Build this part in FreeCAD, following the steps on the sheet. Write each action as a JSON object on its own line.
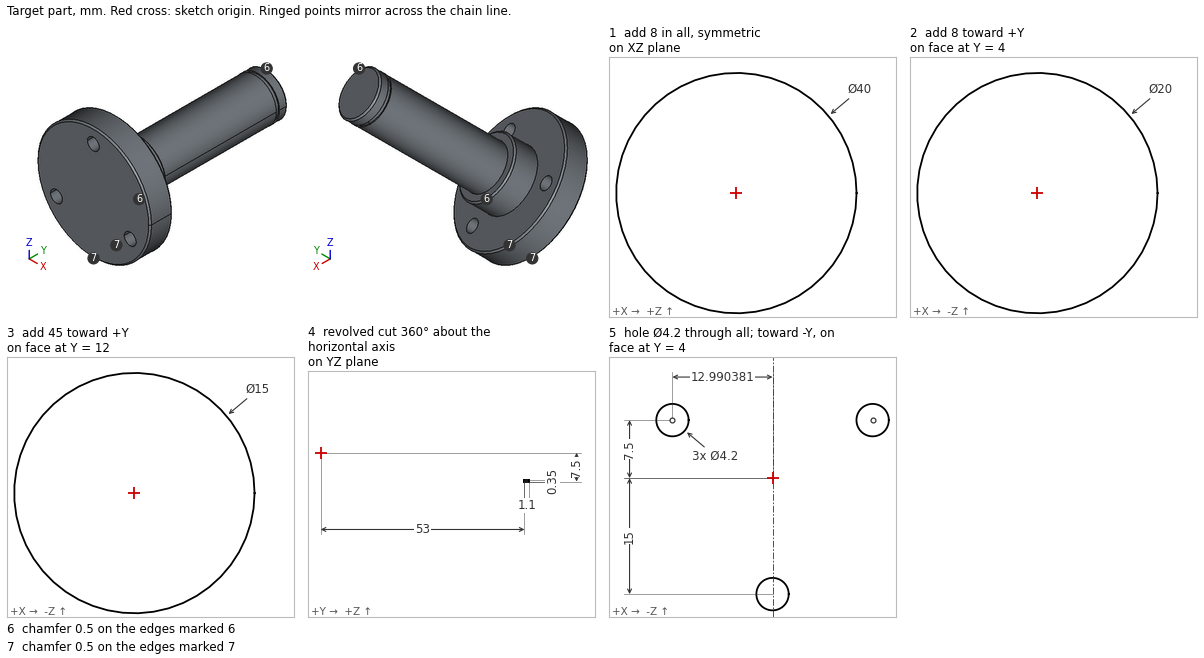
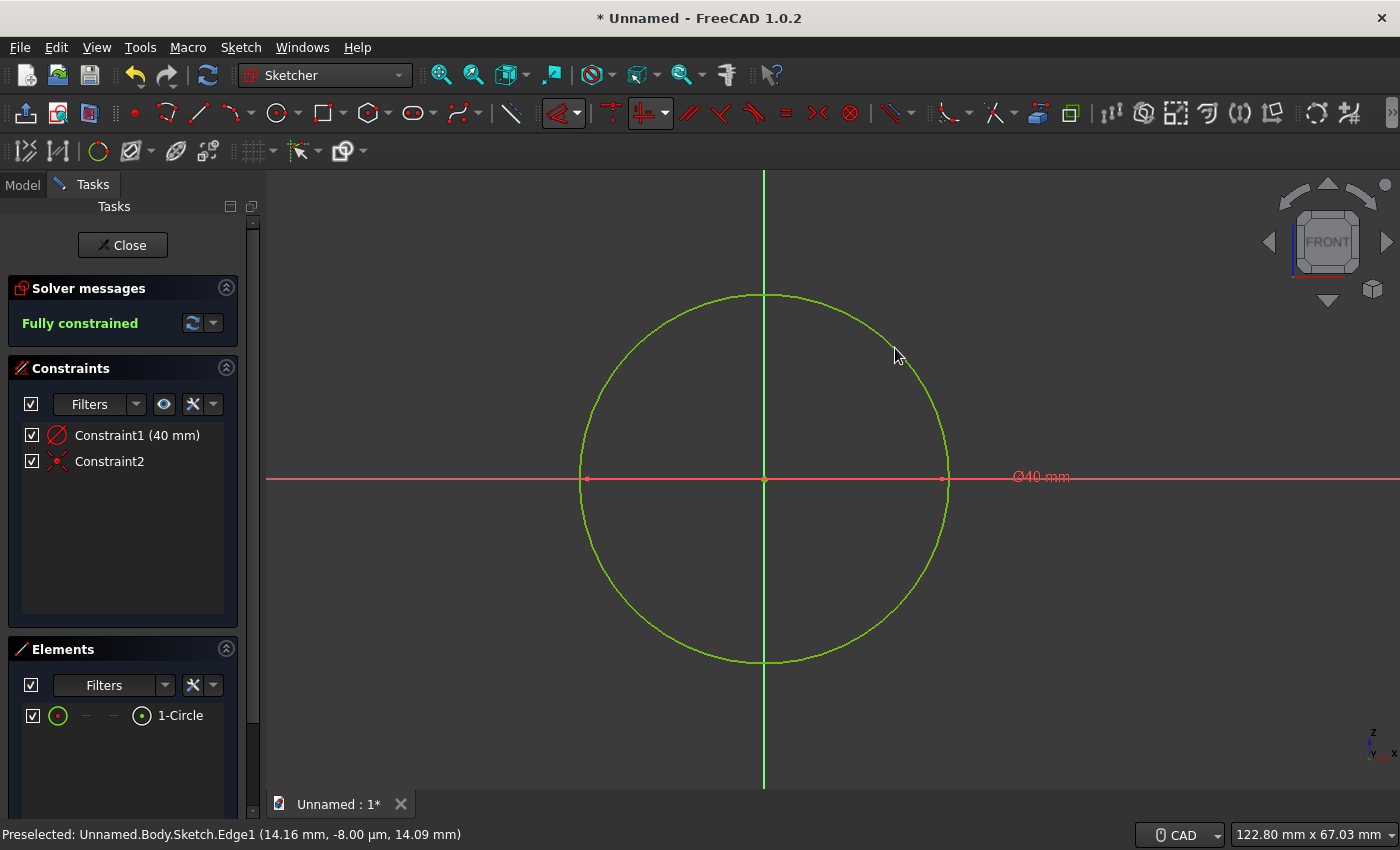
{"action": "left_click", "coordinate": [123, 245]}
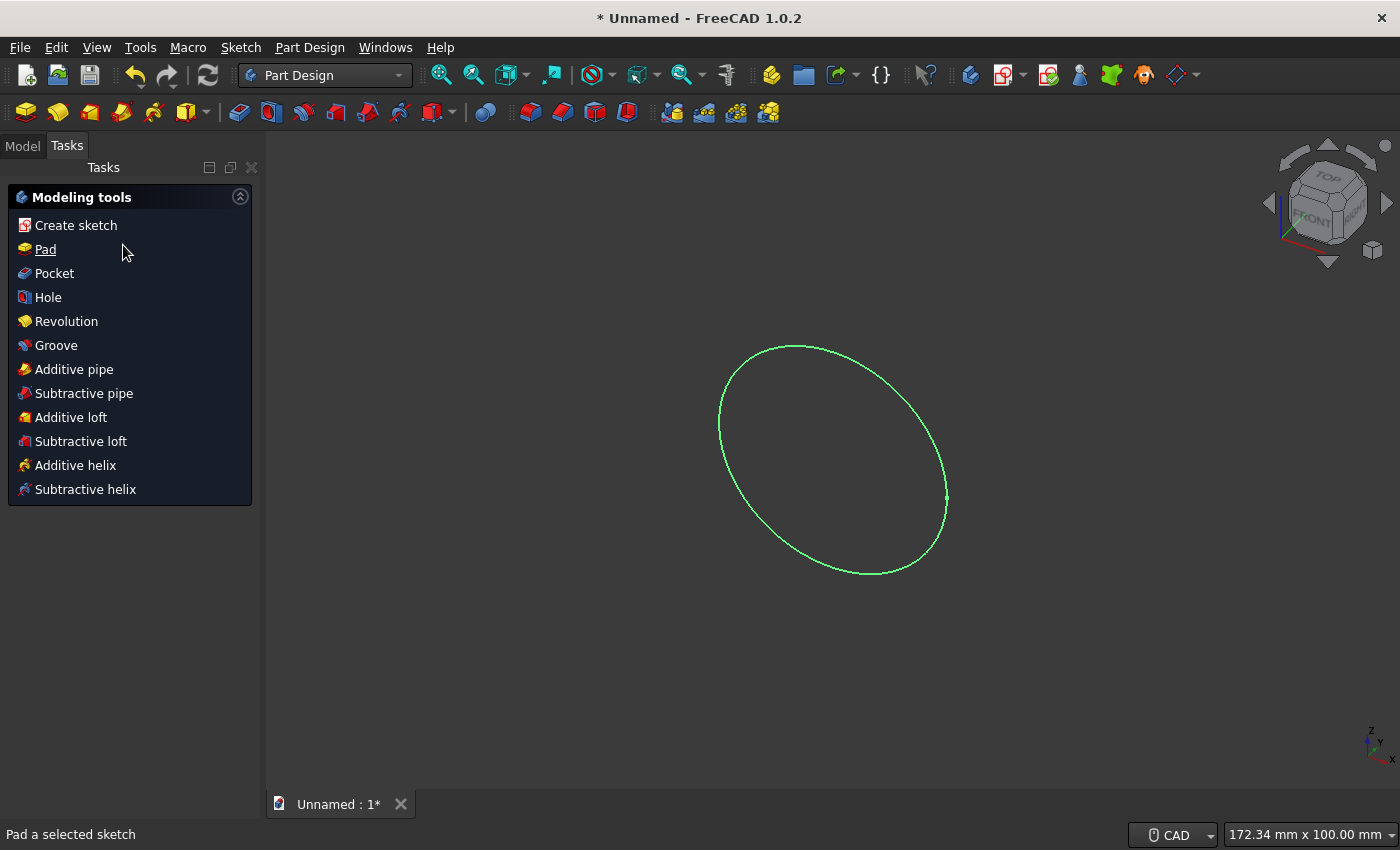
{"action": "left_click", "coordinate": [26, 112]}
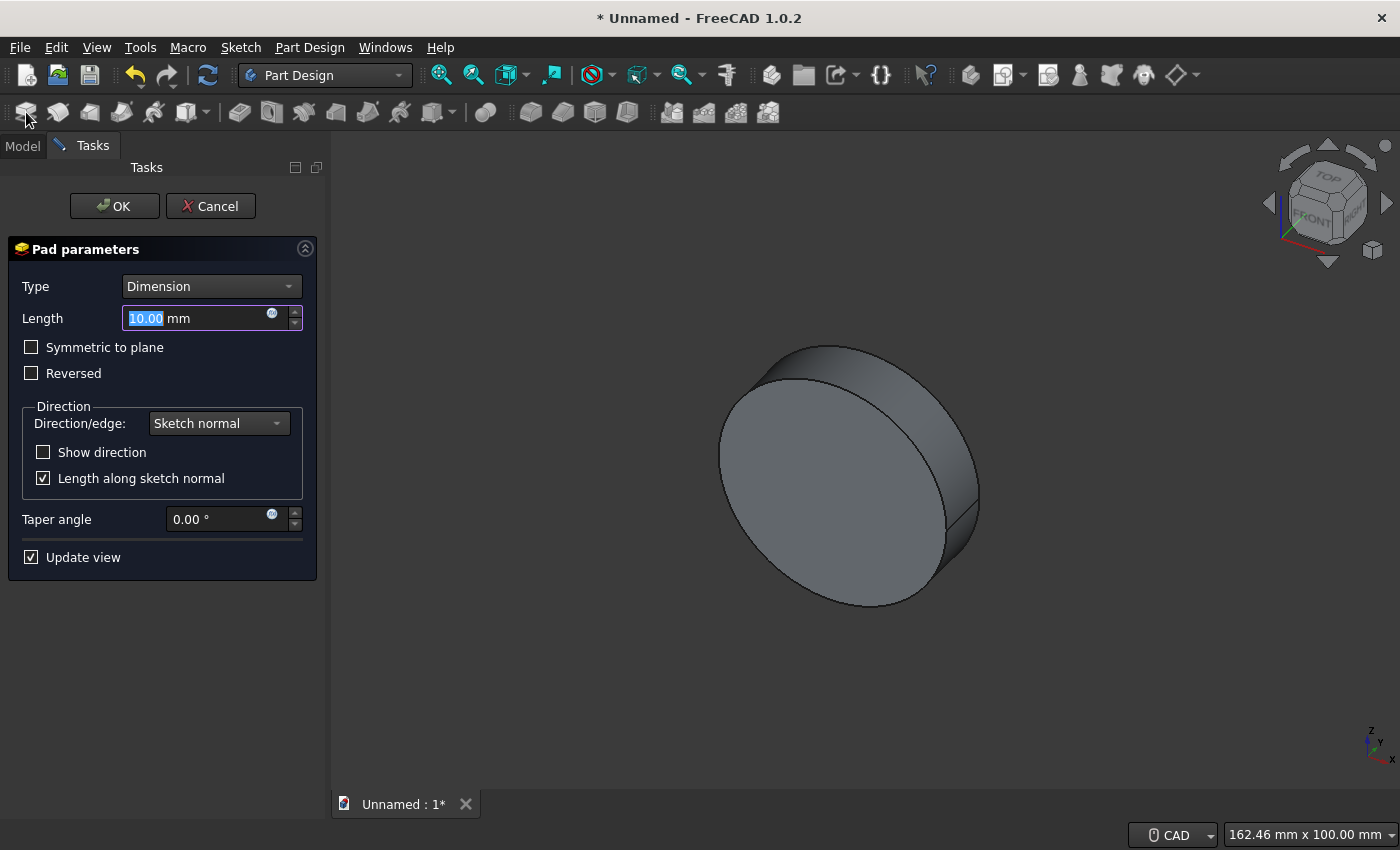
{"action": "type", "text": "8"}
{"action": "key", "text": "Tab"}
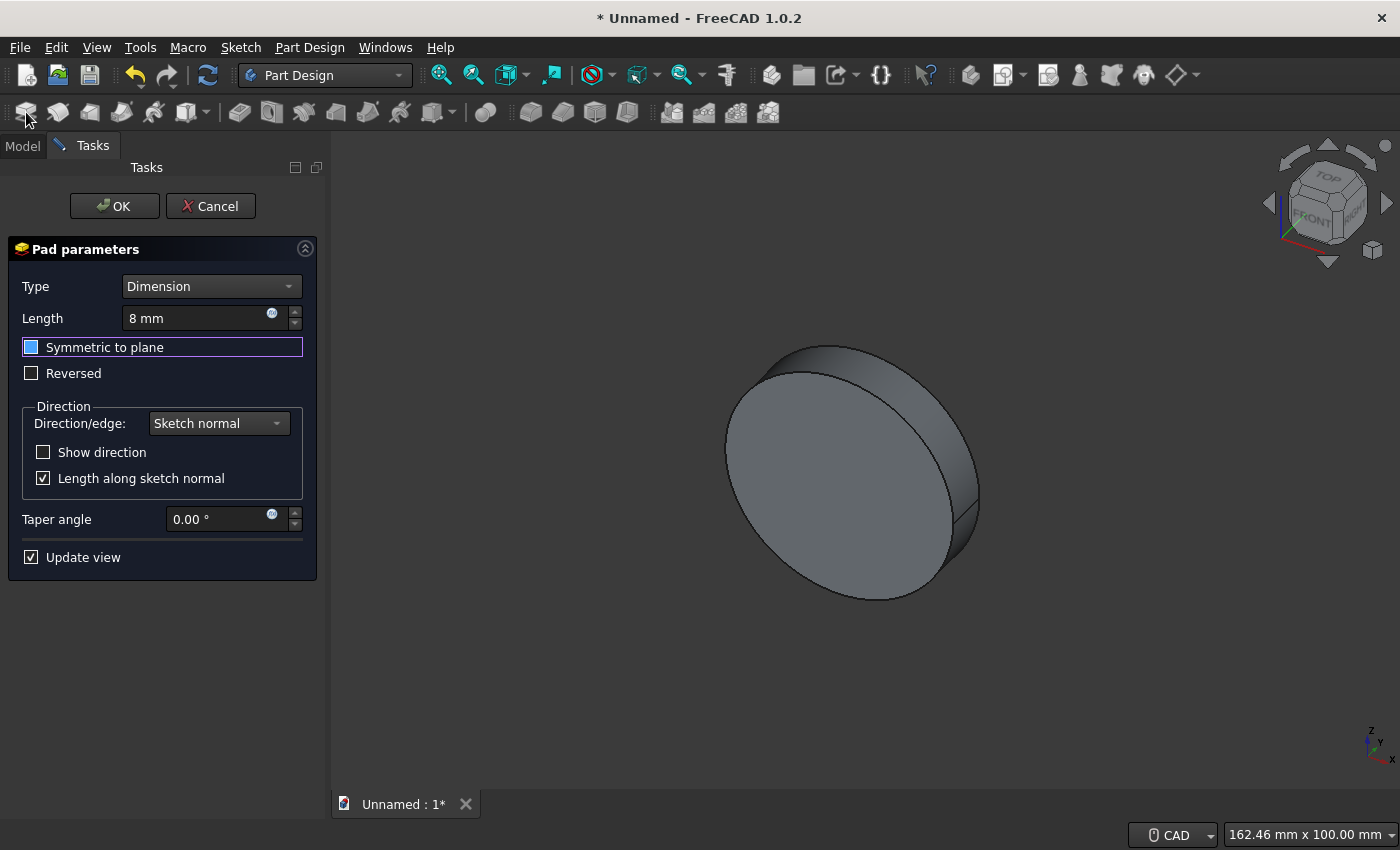
{"action": "left_click", "coordinate": [30, 347]}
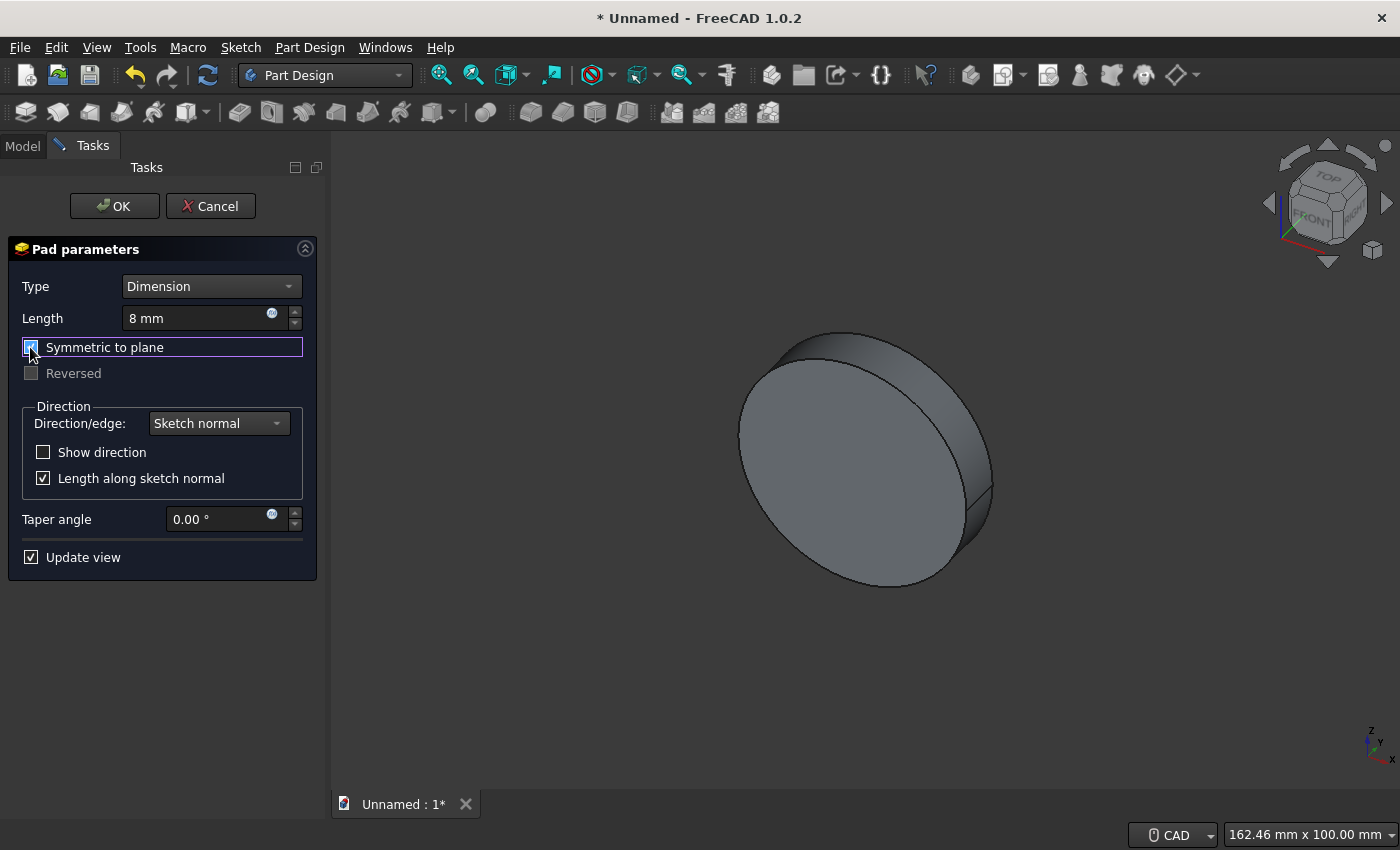
{"action": "left_click", "coordinate": [115, 206]}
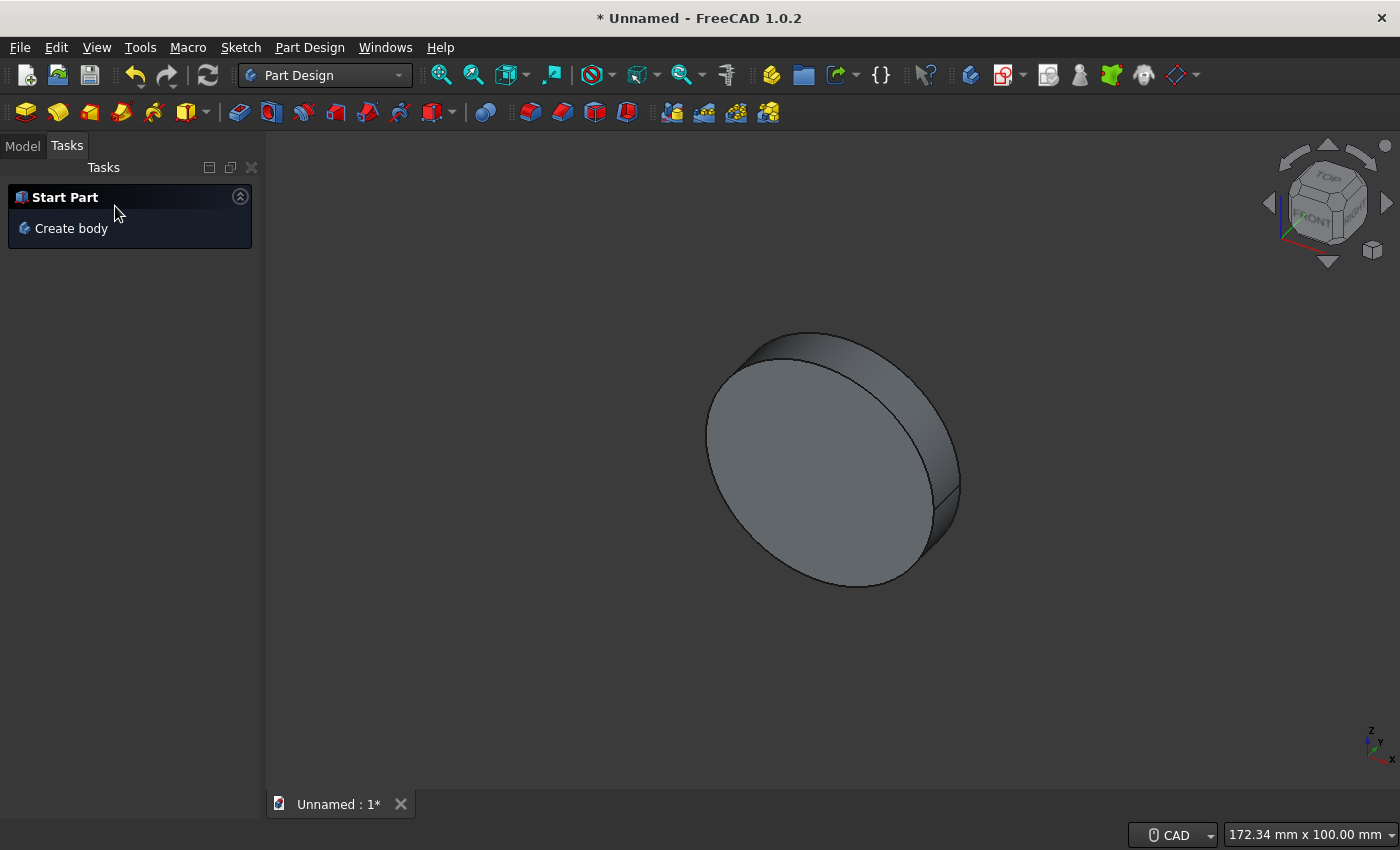
{"action": "key", "text": "4"}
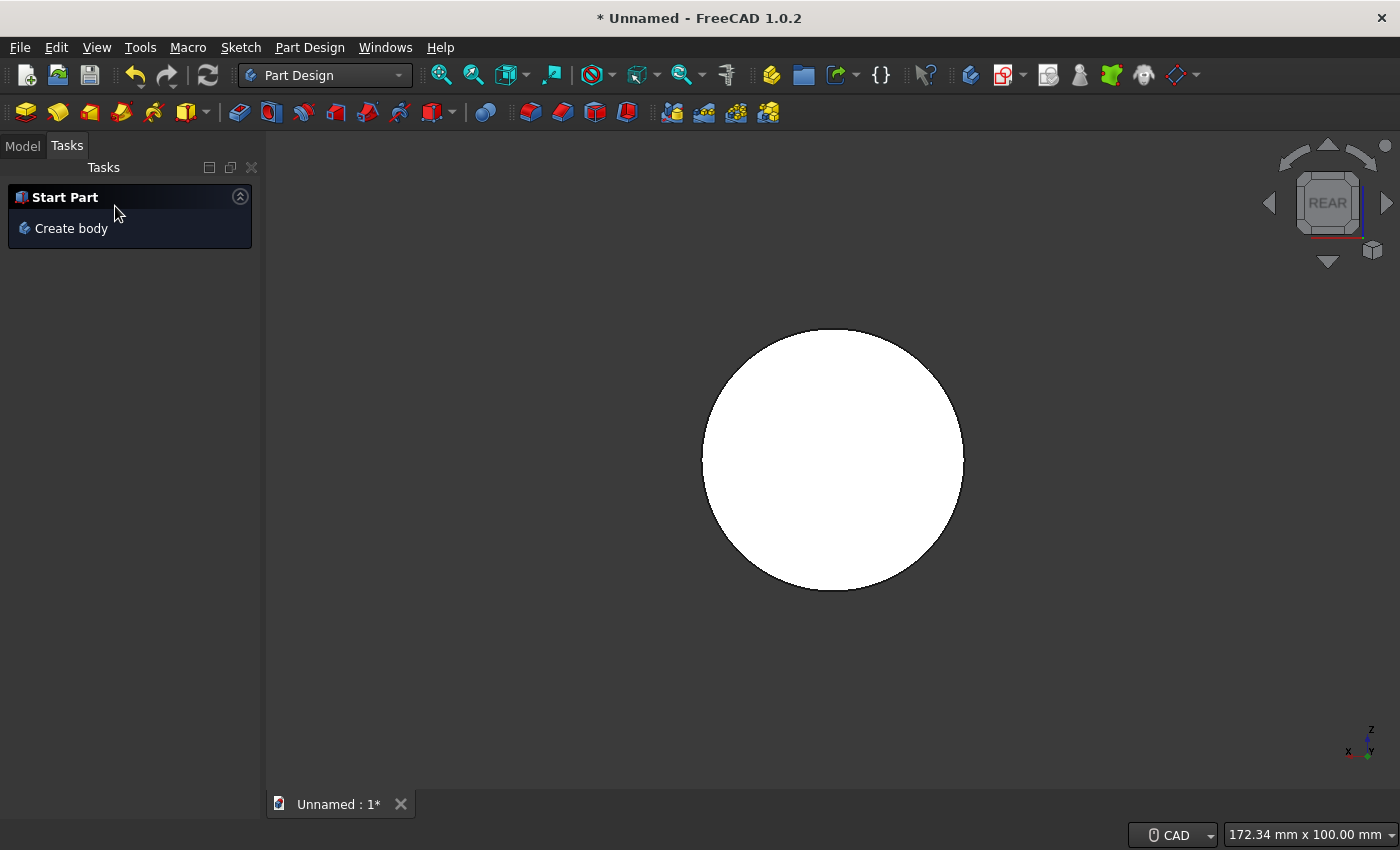
{"action": "left_click", "coordinate": [442, 76]}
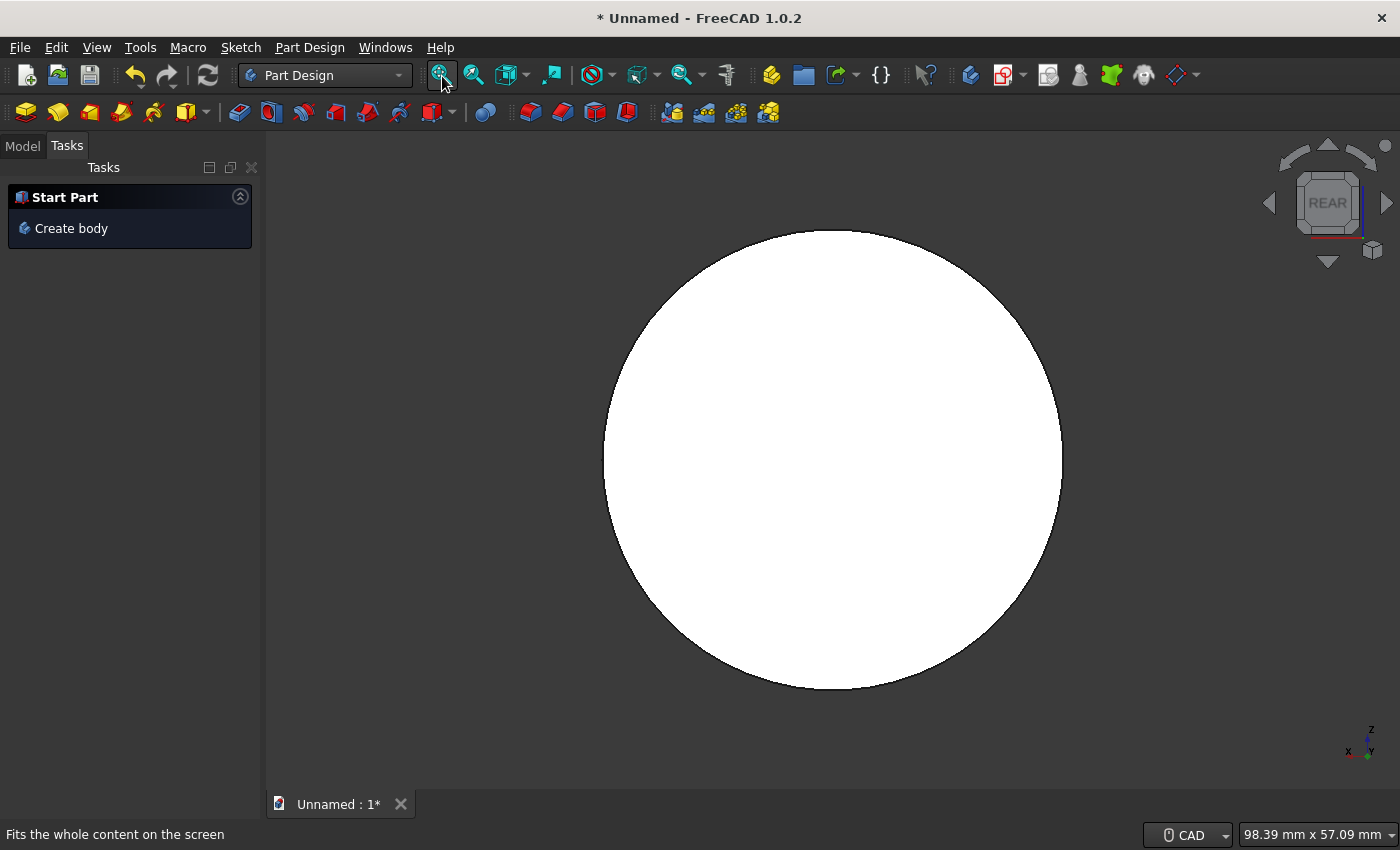
{"action": "left_click", "coordinate": [833, 459]}